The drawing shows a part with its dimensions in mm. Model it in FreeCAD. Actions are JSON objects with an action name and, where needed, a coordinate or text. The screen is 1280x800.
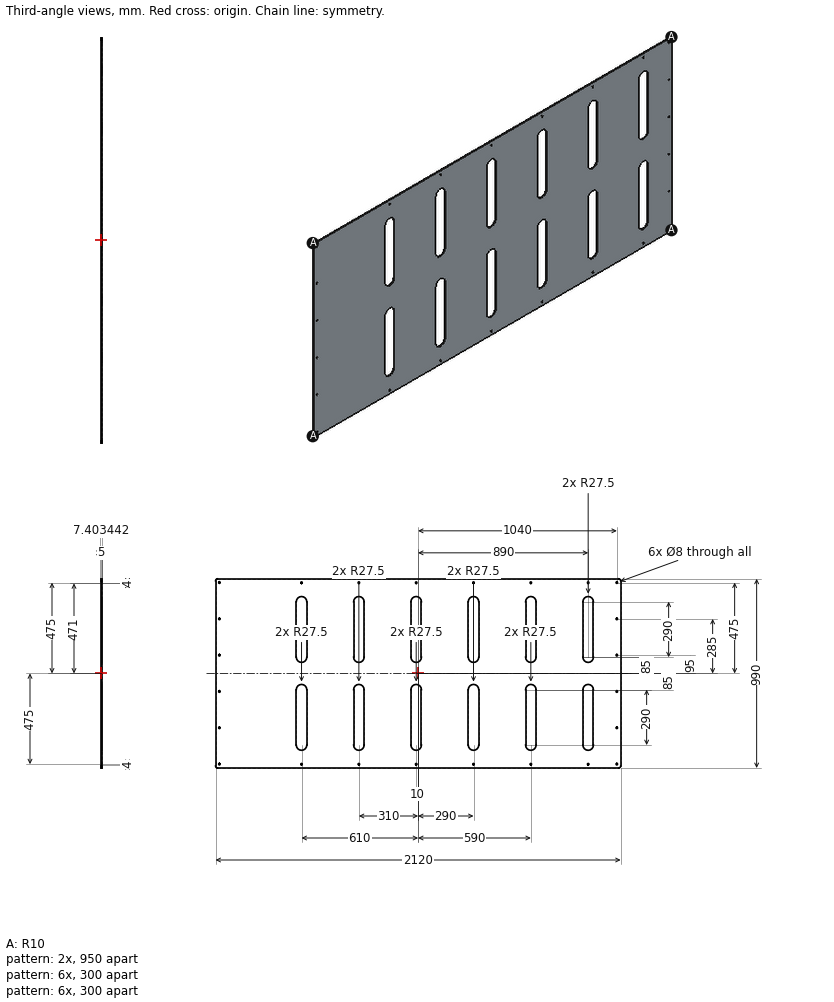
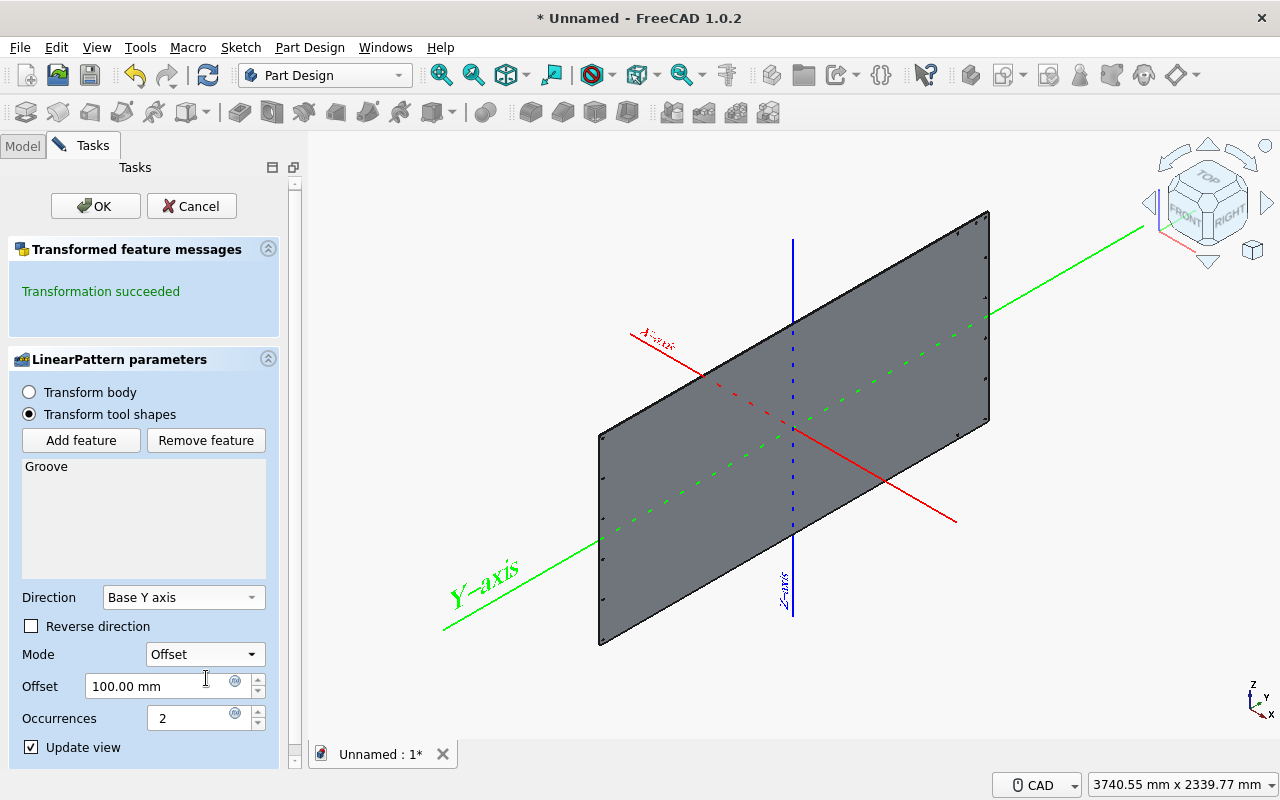
{"action": "triple_click", "coordinate": [168, 686]}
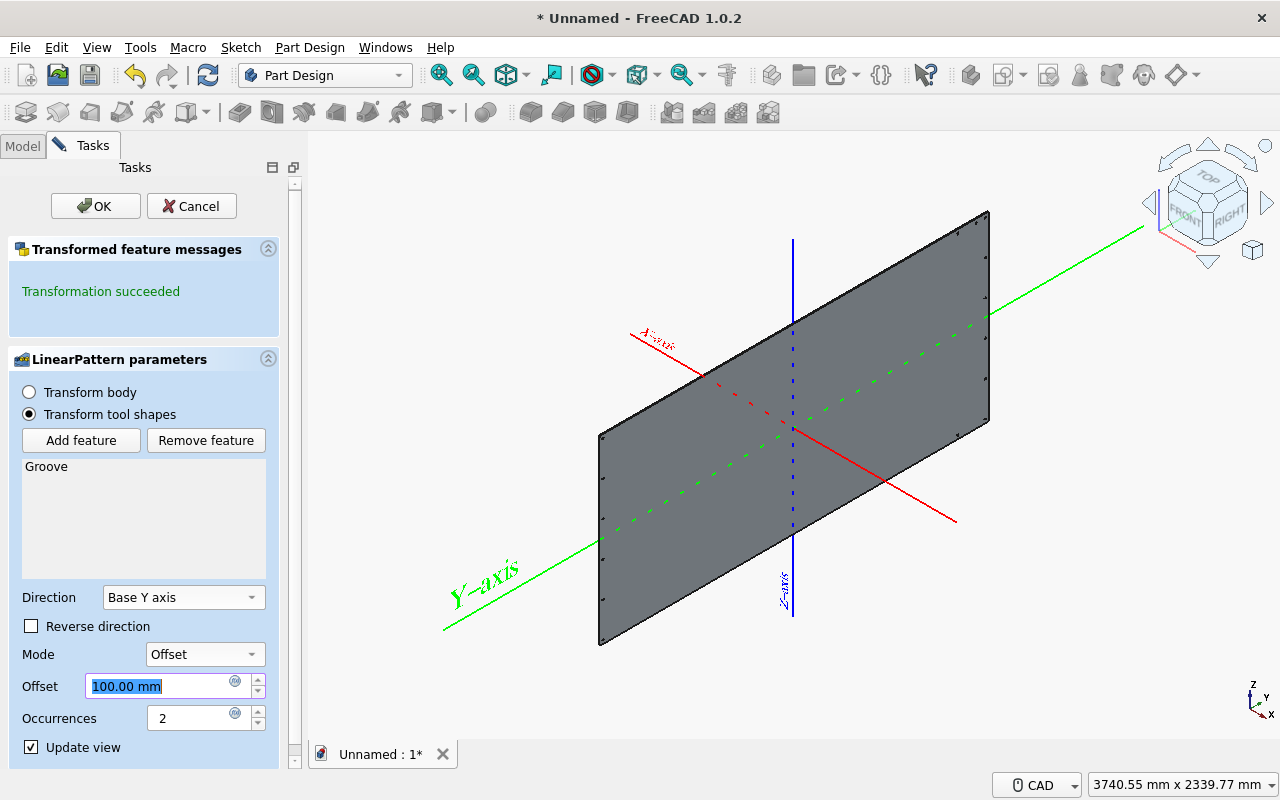
{"action": "type", "text": "300"}
{"action": "key", "text": "Tab"}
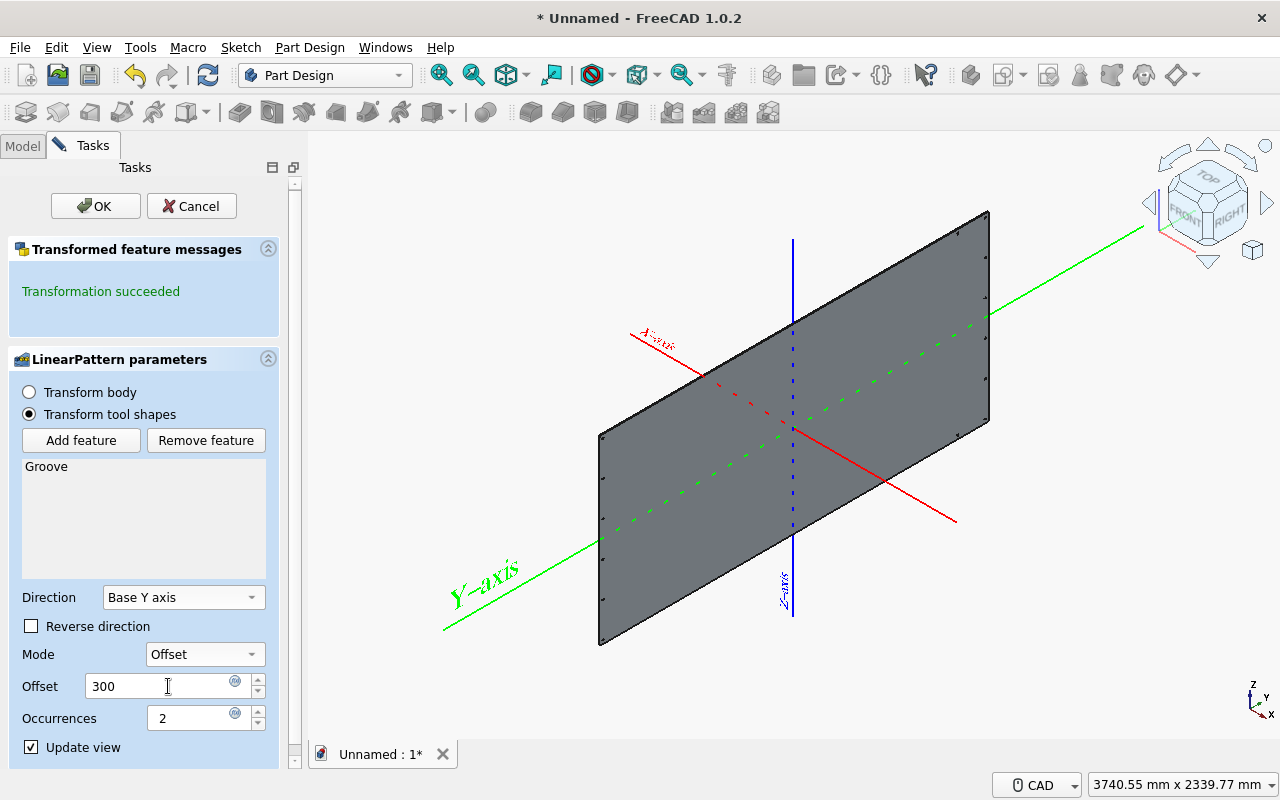
{"action": "triple_click", "coordinate": [198, 718]}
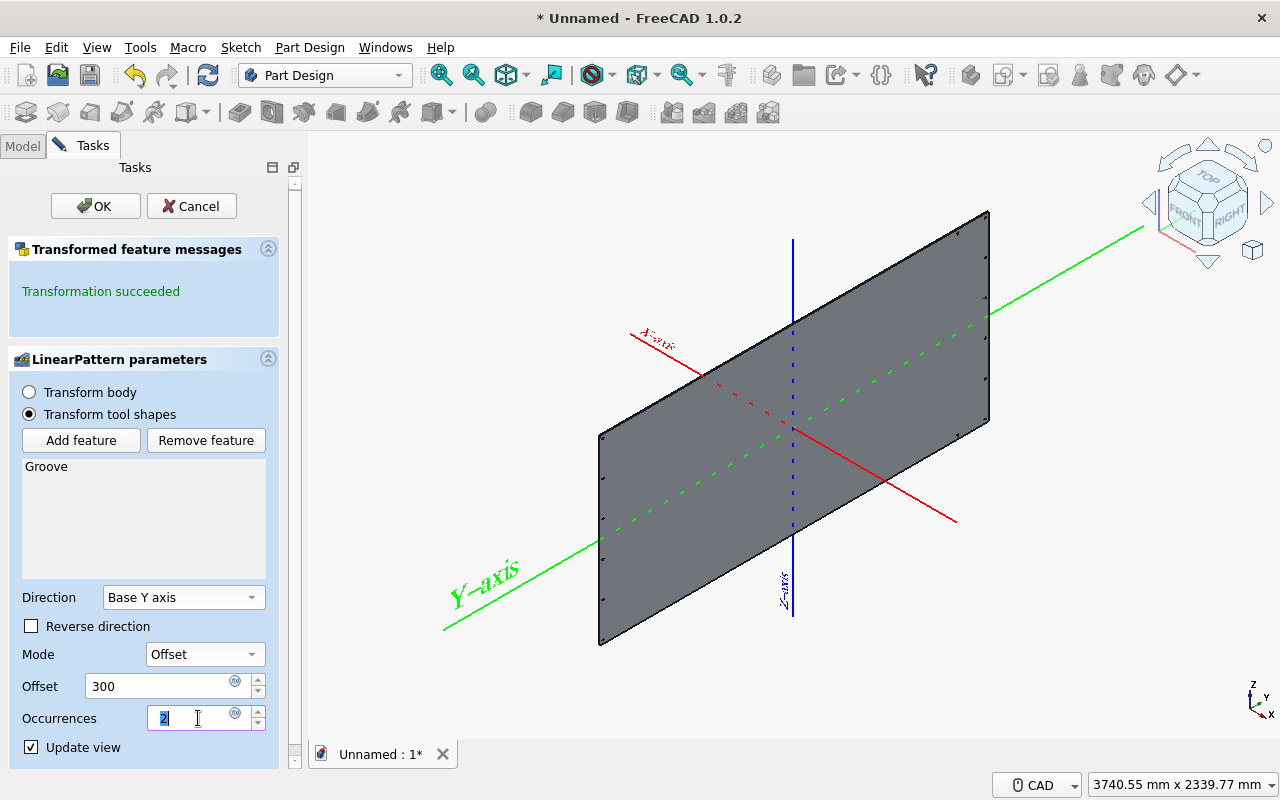
{"action": "type", "text": "6"}
{"action": "key", "text": "Tab"}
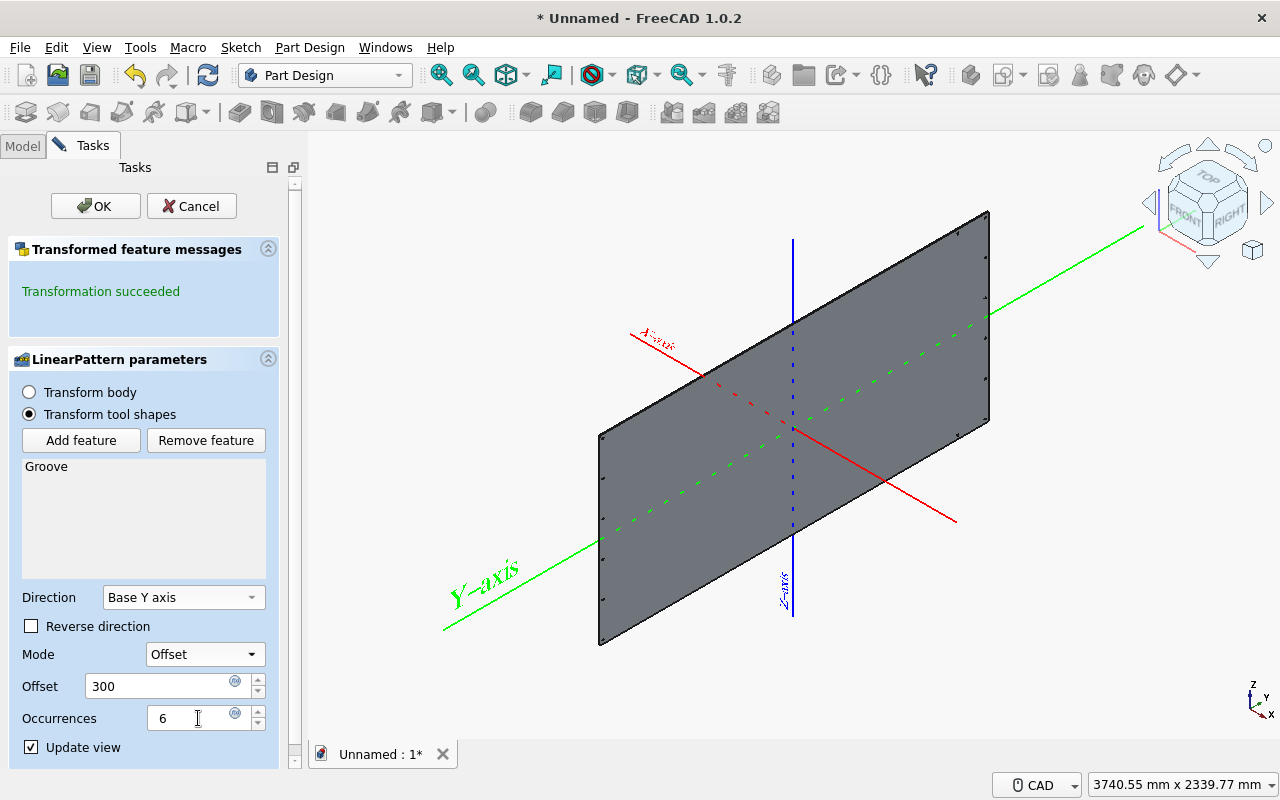
{"action": "left_click", "coordinate": [30, 626]}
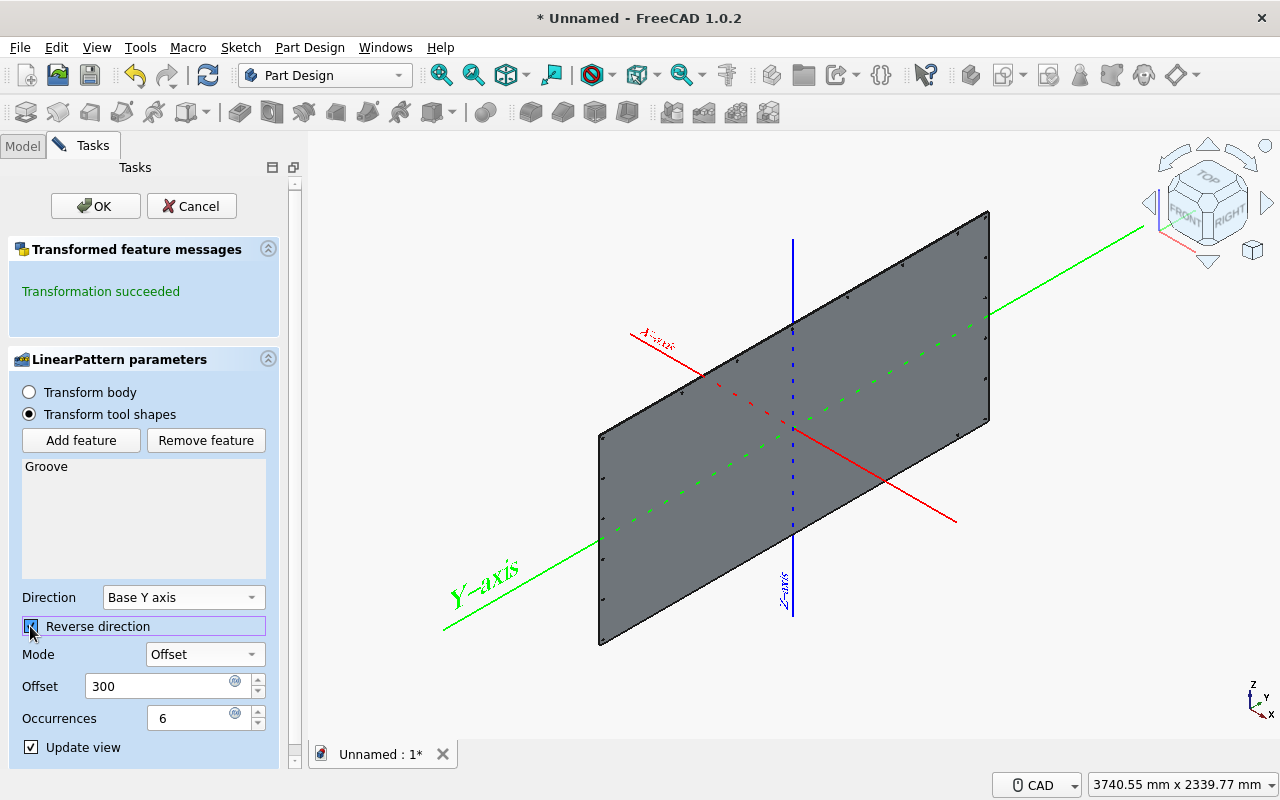
{"action": "left_click", "coordinate": [96, 206]}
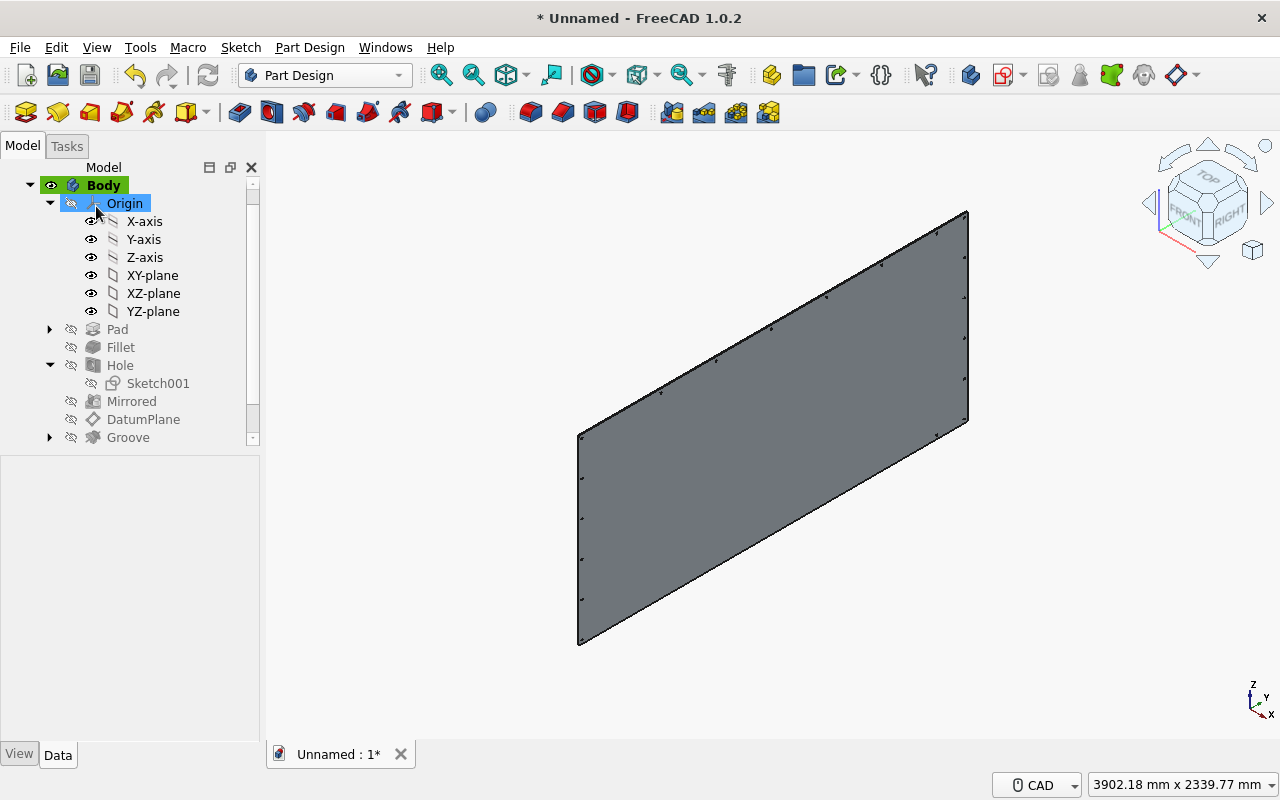
{"action": "left_click", "coordinate": [136, 293]}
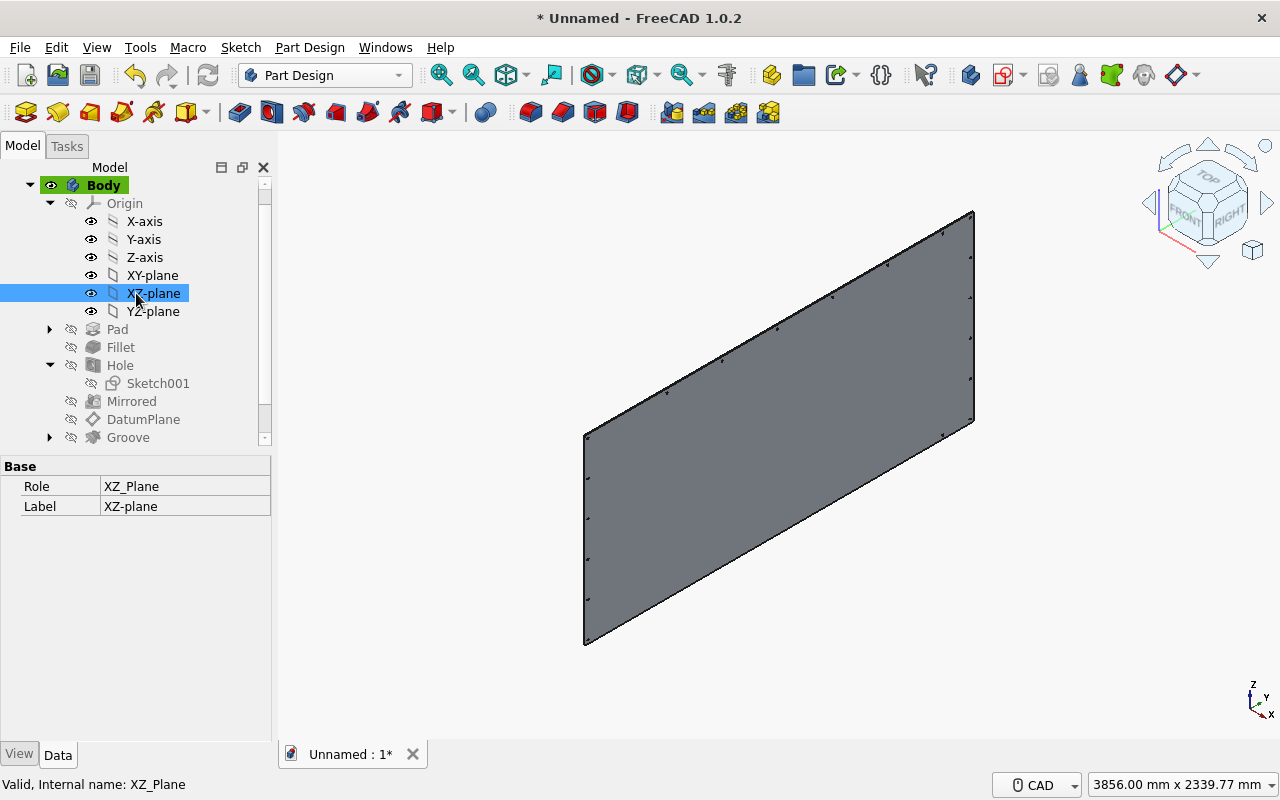
{"action": "left_click", "coordinate": [1176, 76]}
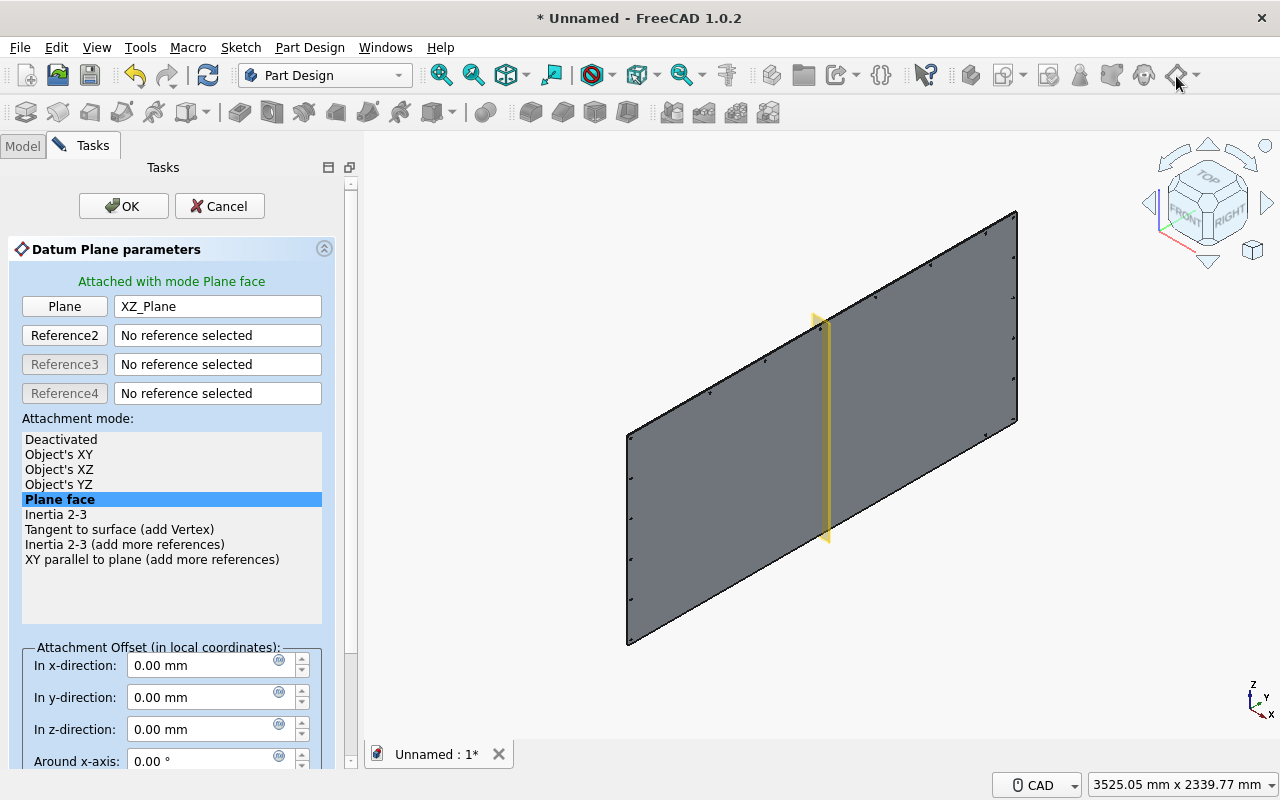
{"action": "triple_click", "coordinate": [210, 729]}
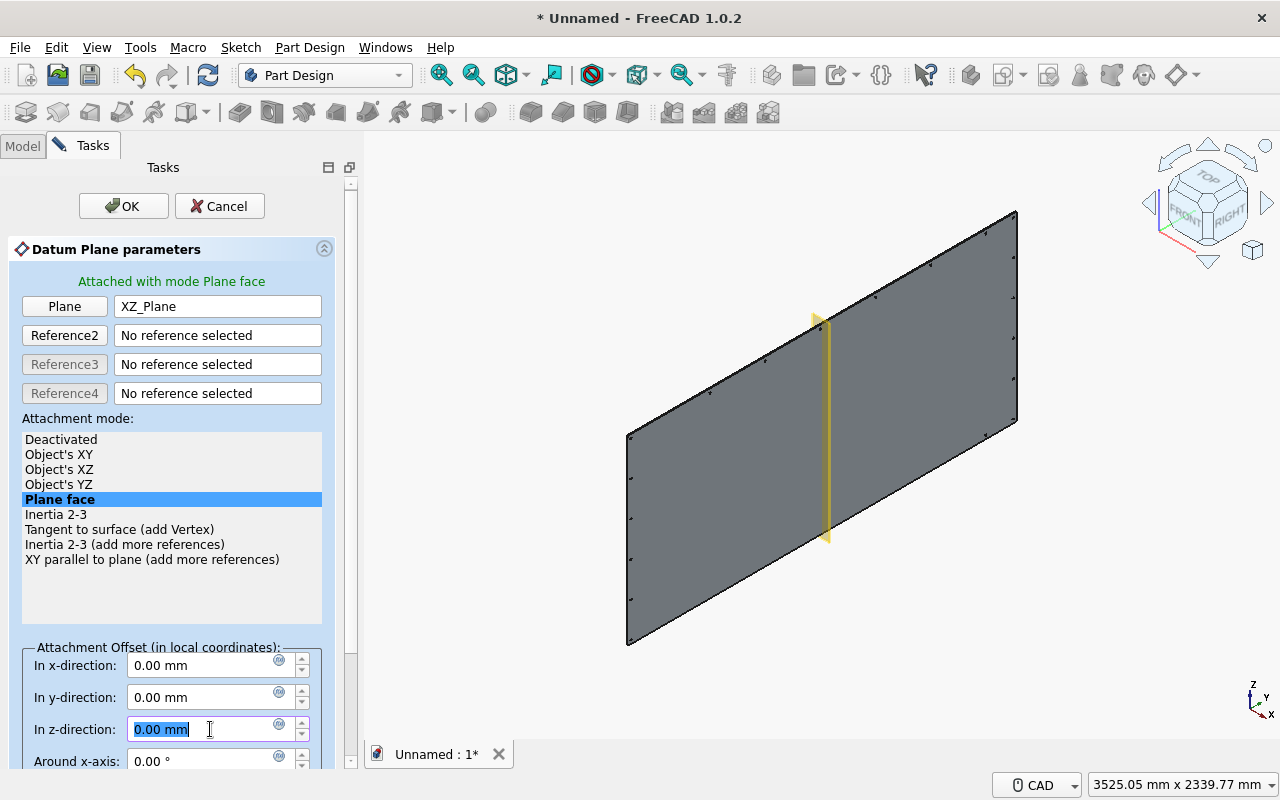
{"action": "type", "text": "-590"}
{"action": "key", "text": "Tab"}